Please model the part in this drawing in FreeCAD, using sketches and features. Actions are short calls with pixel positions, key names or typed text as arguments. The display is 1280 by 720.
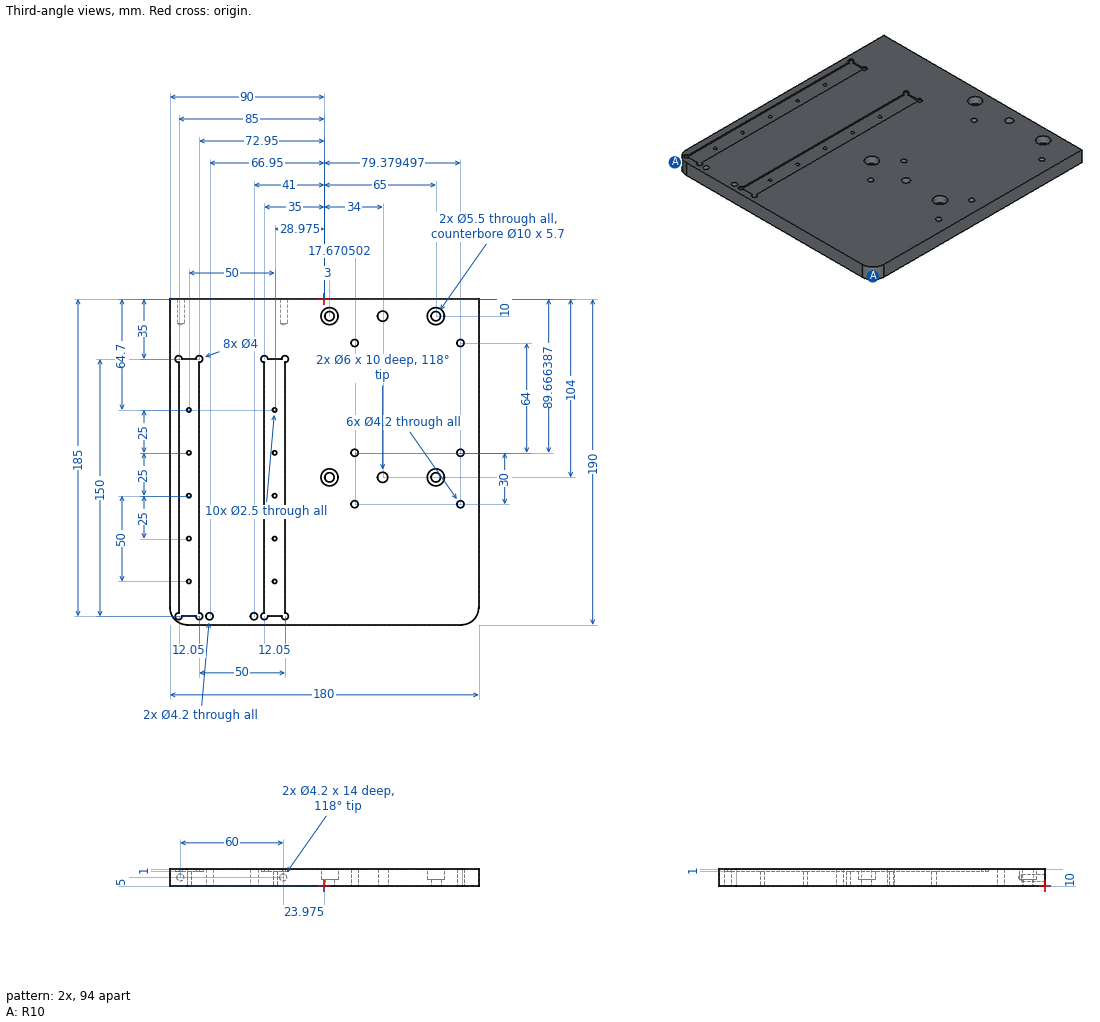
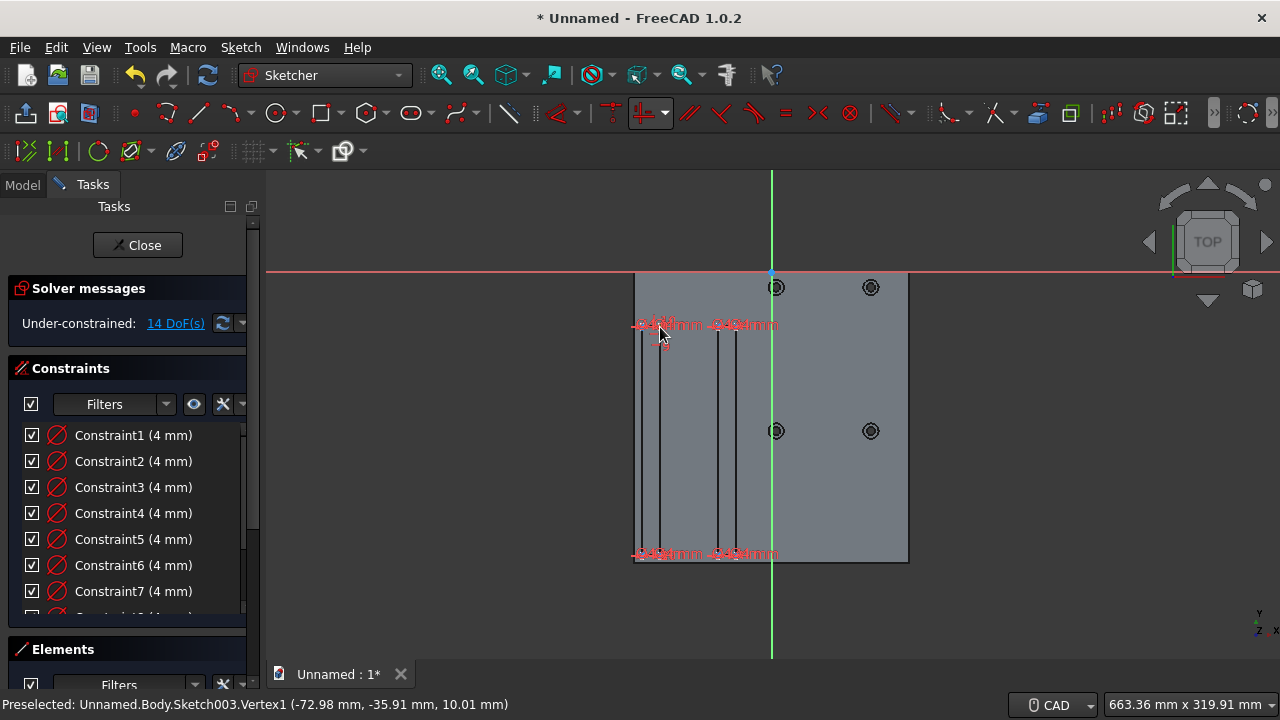
scroll(660, 556, up, 4)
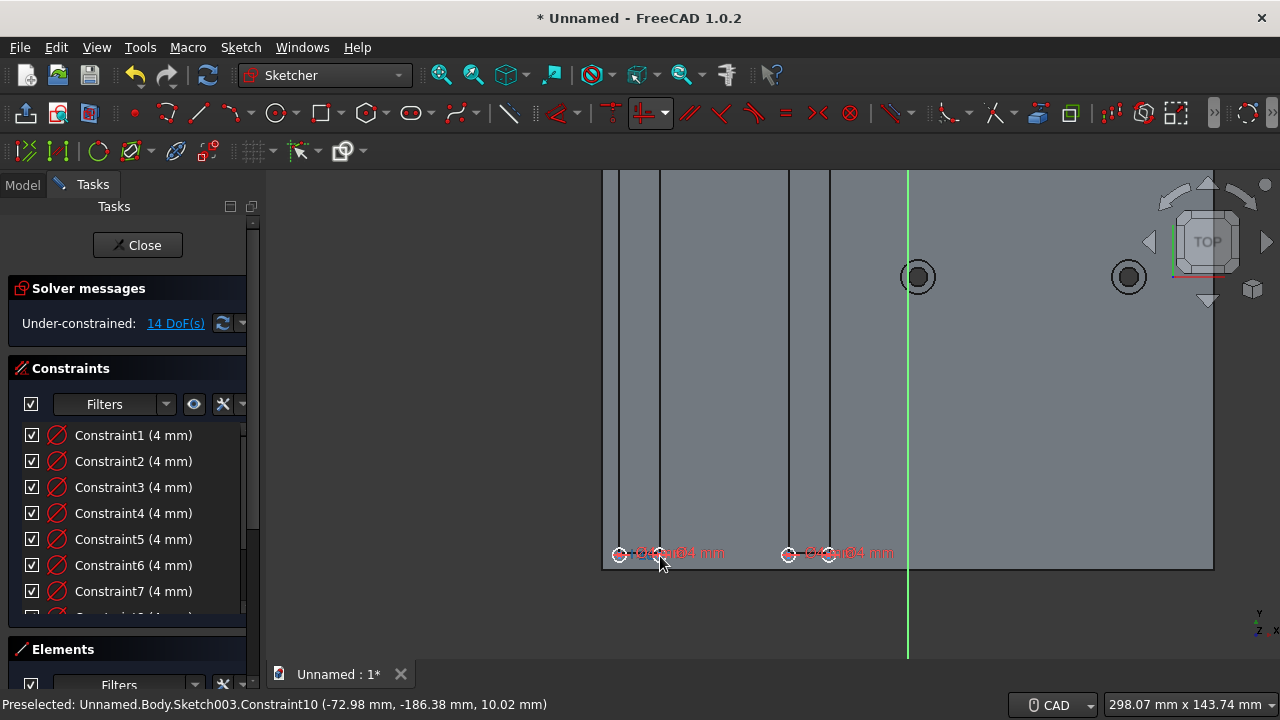
click(660, 555)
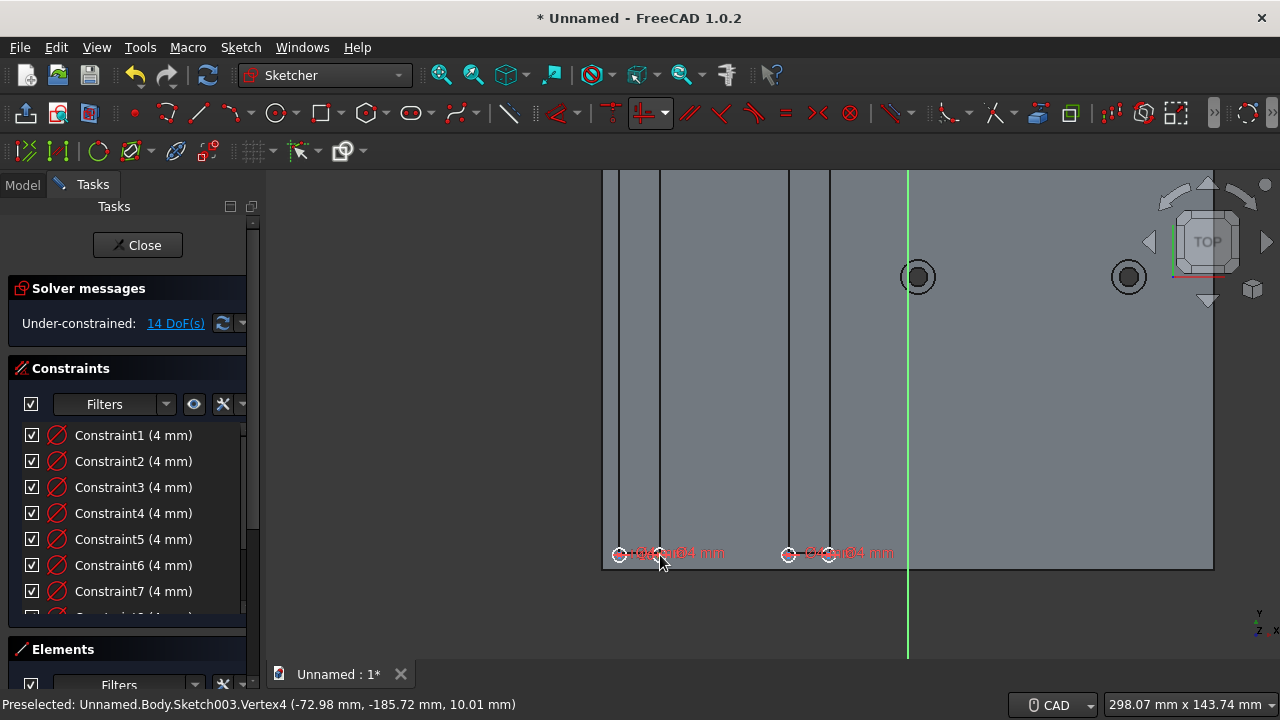
key(v)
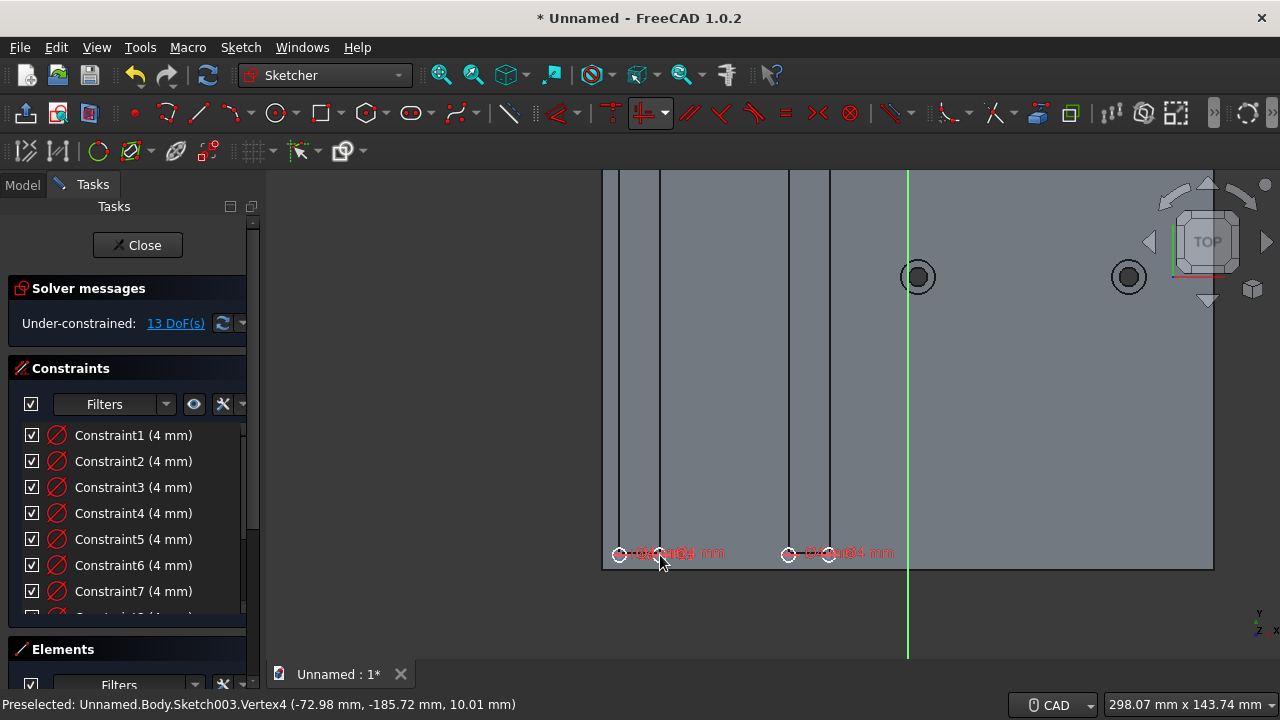
click(619, 555)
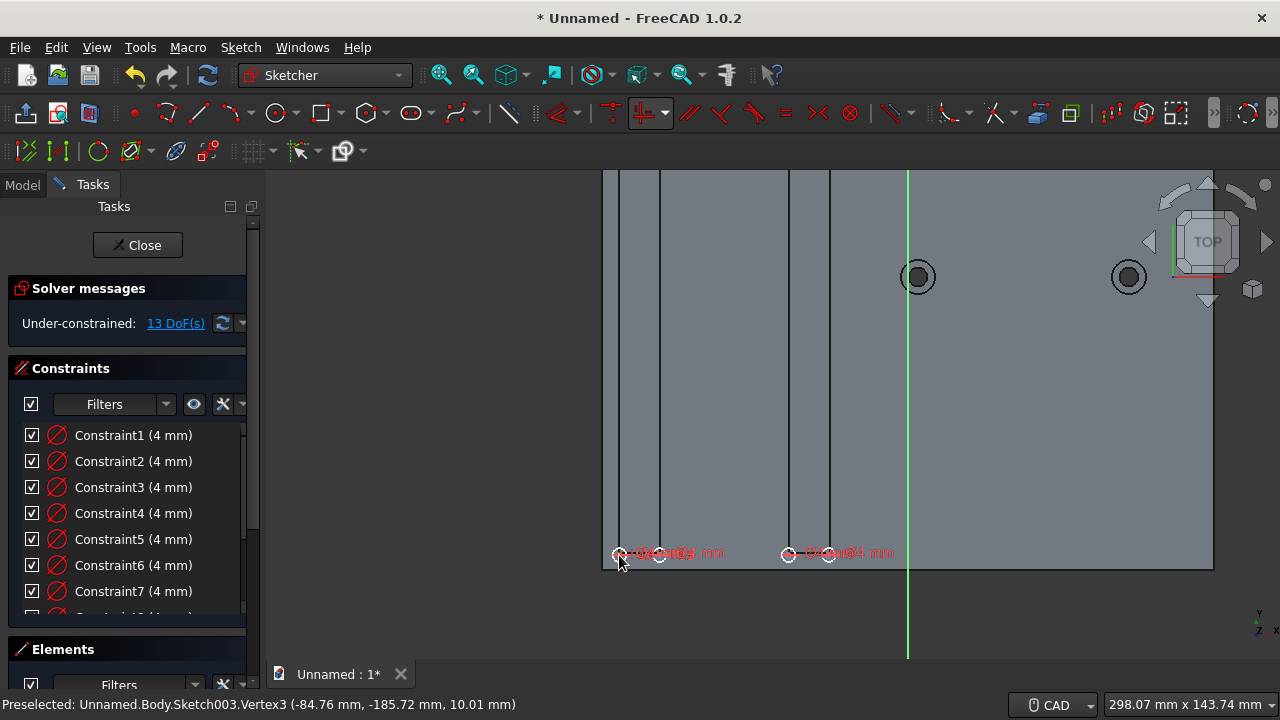
click(660, 555)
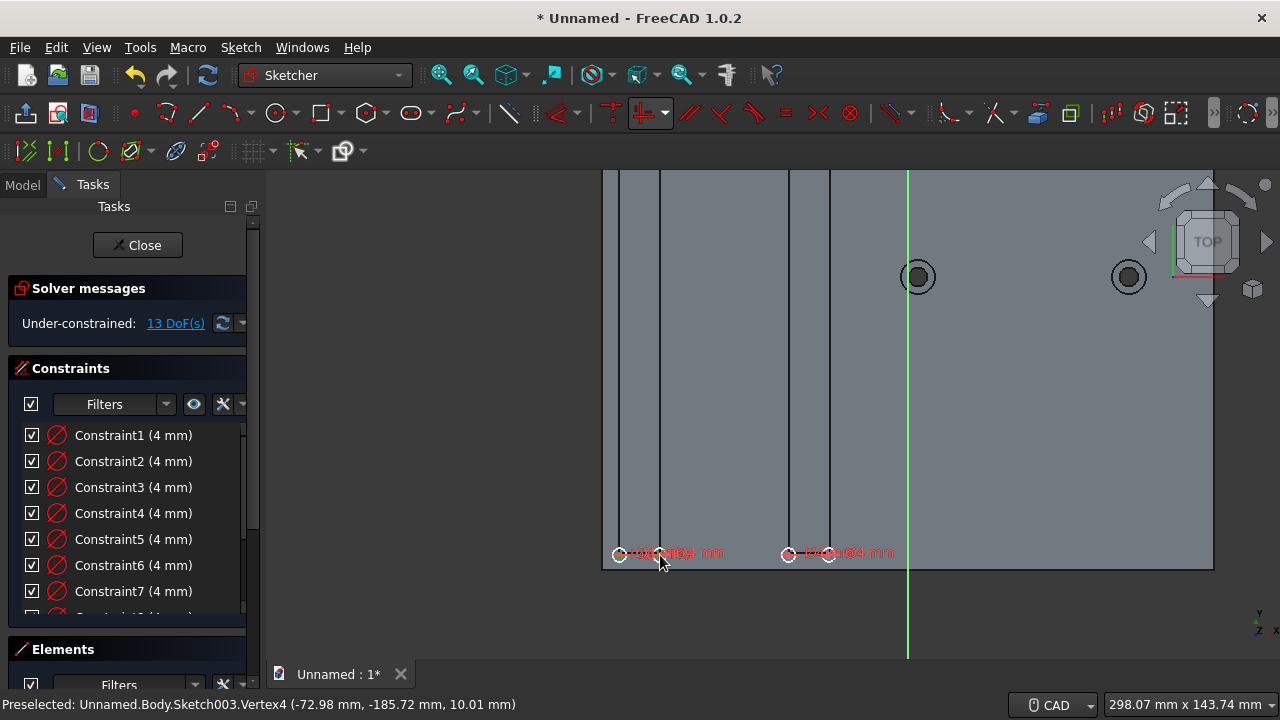
key(h)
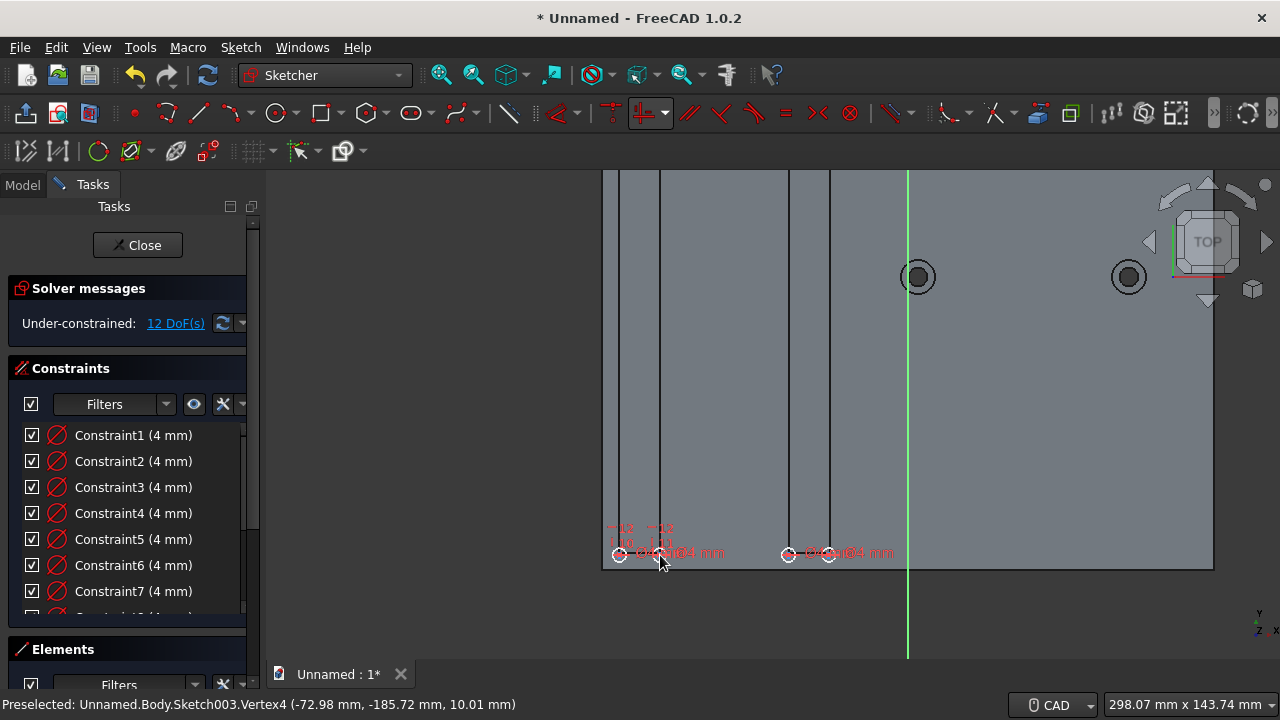
click(660, 555)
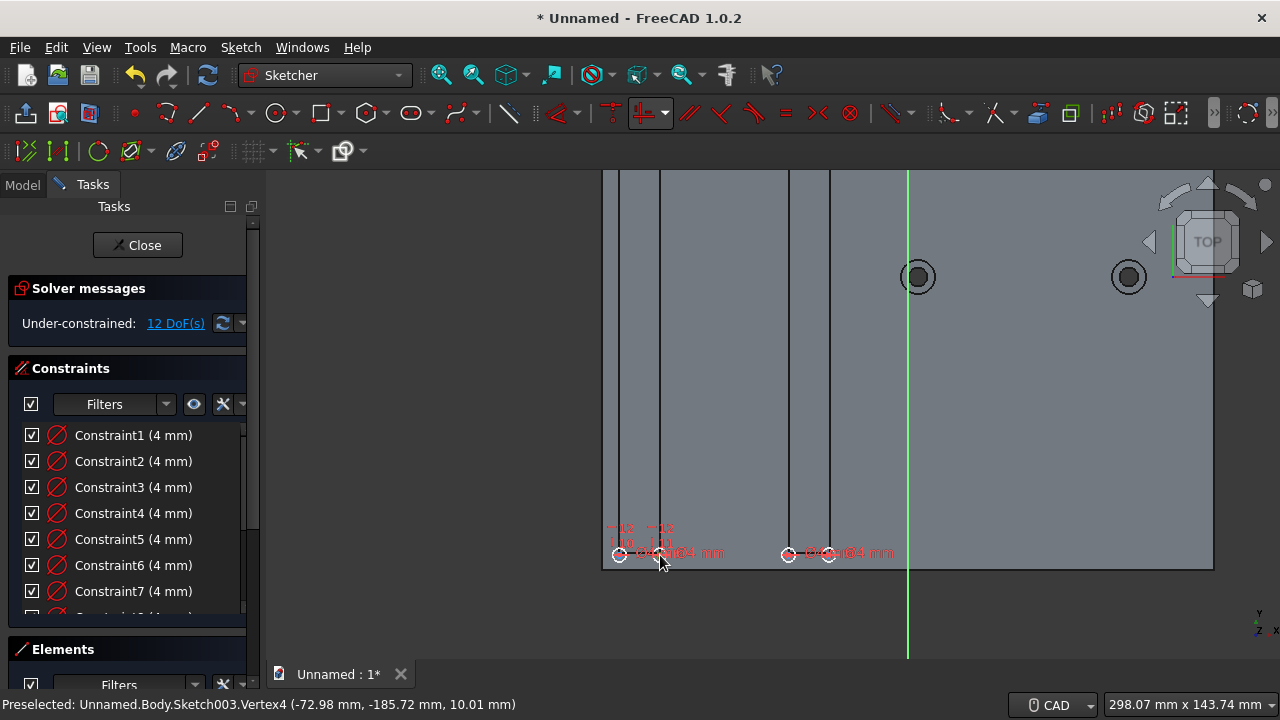
click(789, 555)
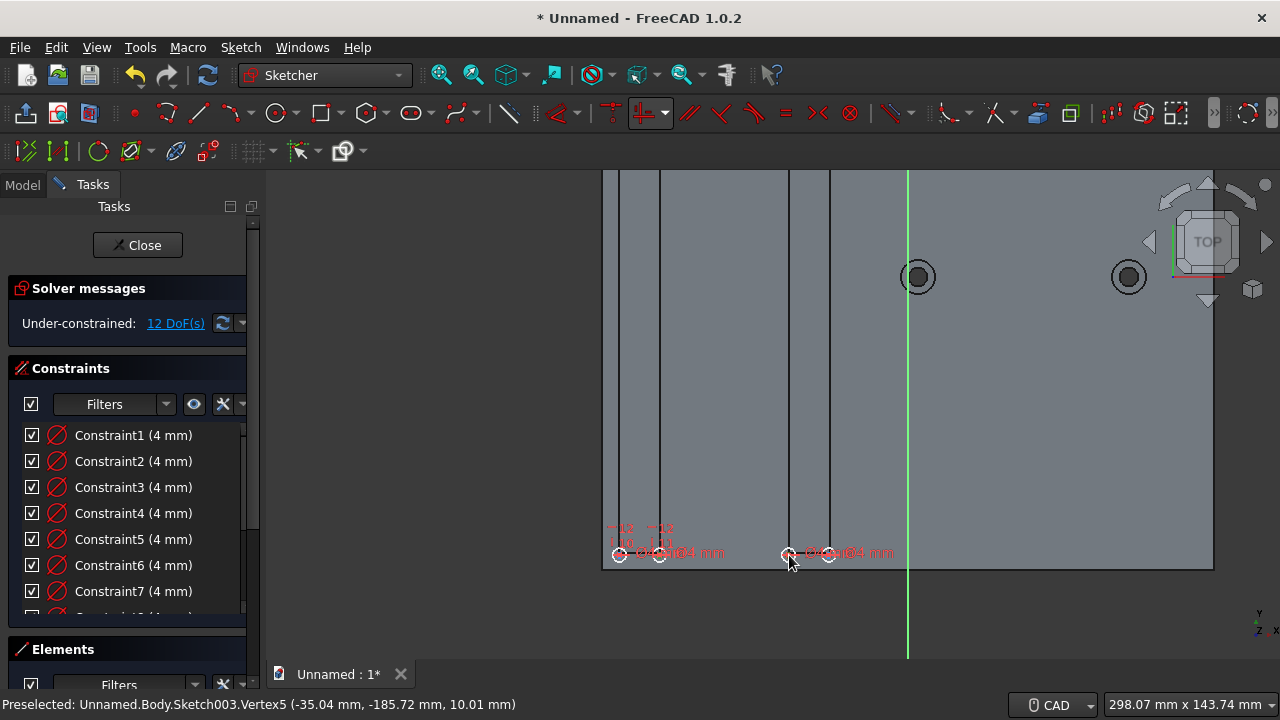
click(668, 114)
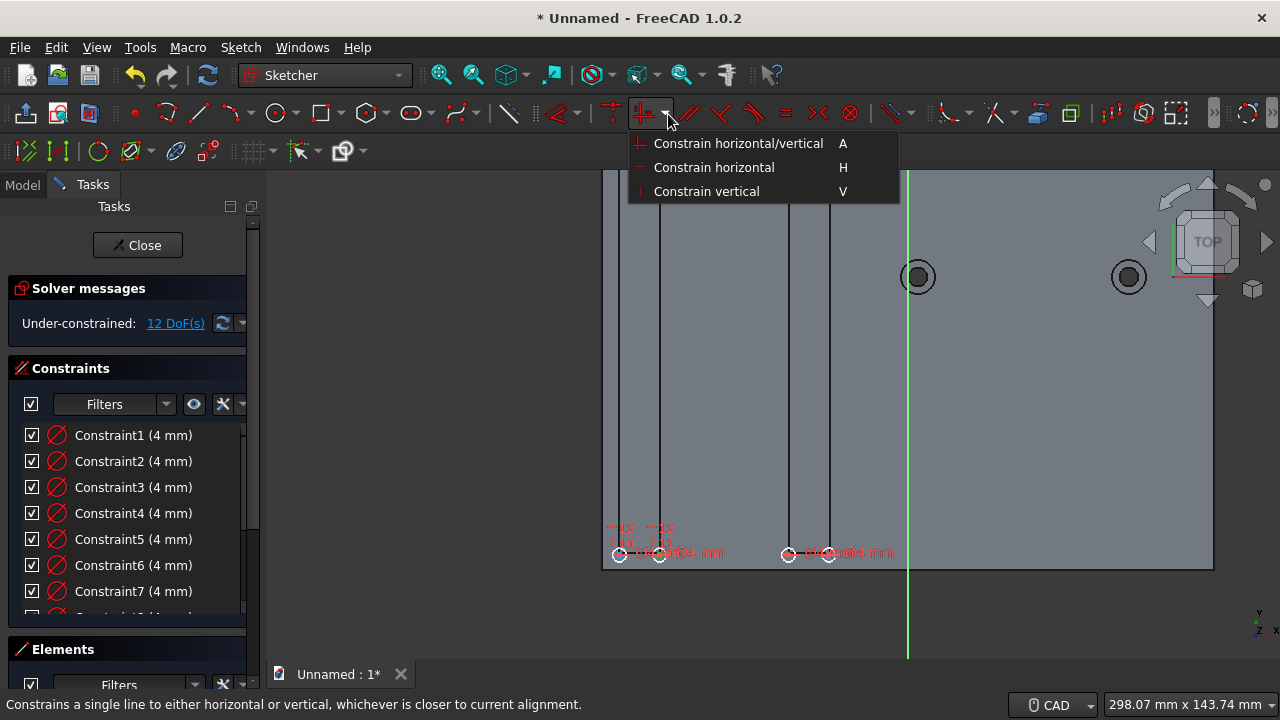
click(764, 167)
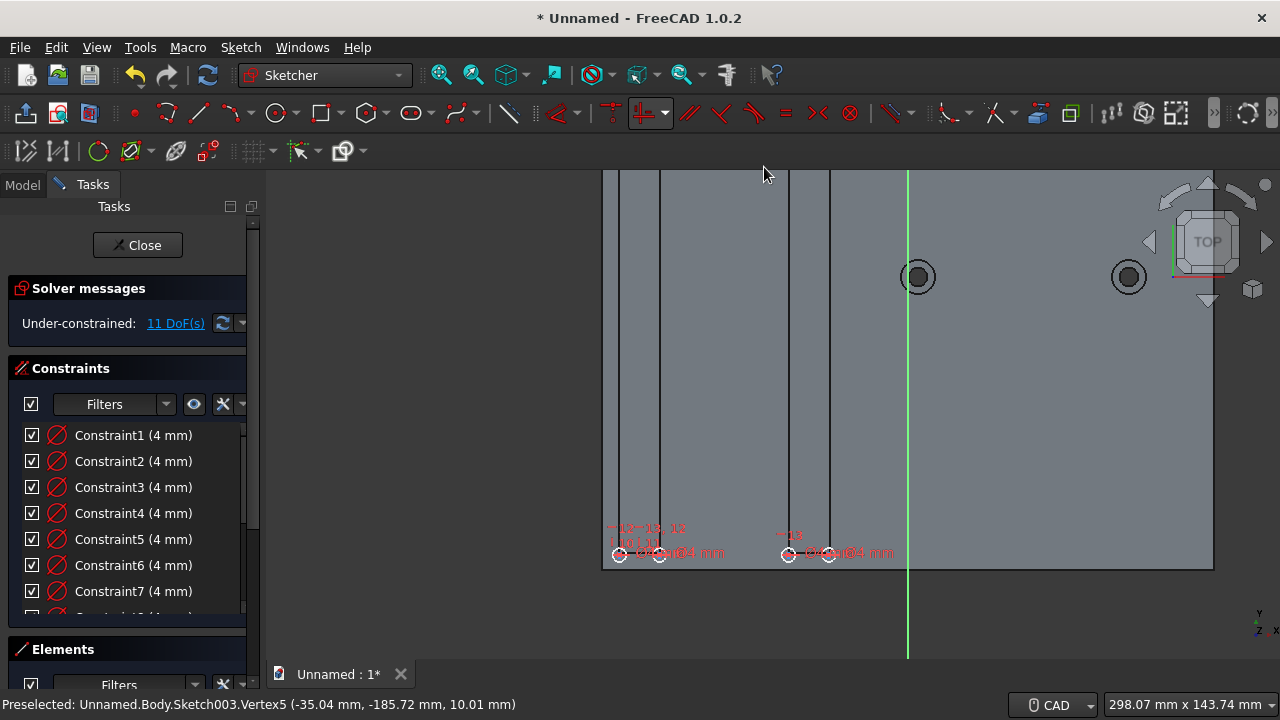
click(789, 555)